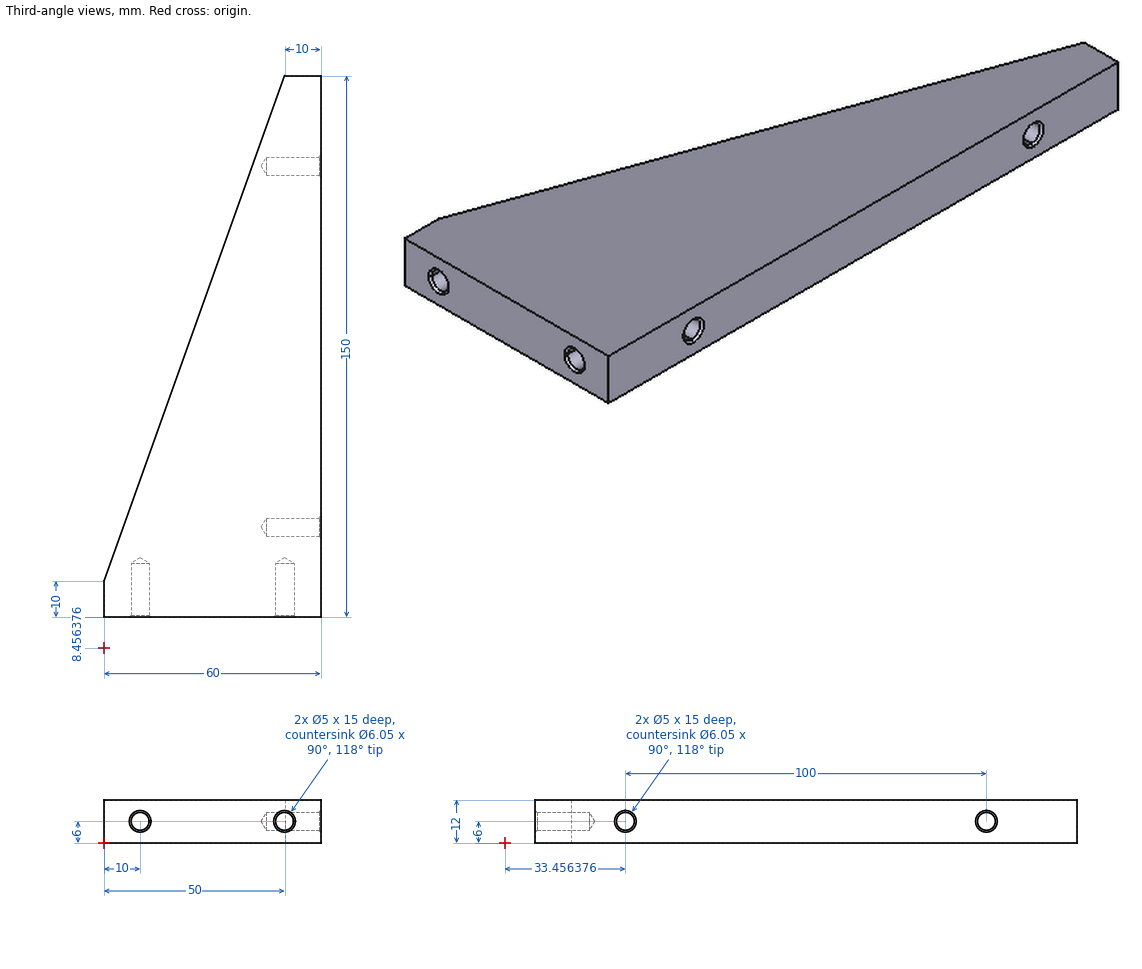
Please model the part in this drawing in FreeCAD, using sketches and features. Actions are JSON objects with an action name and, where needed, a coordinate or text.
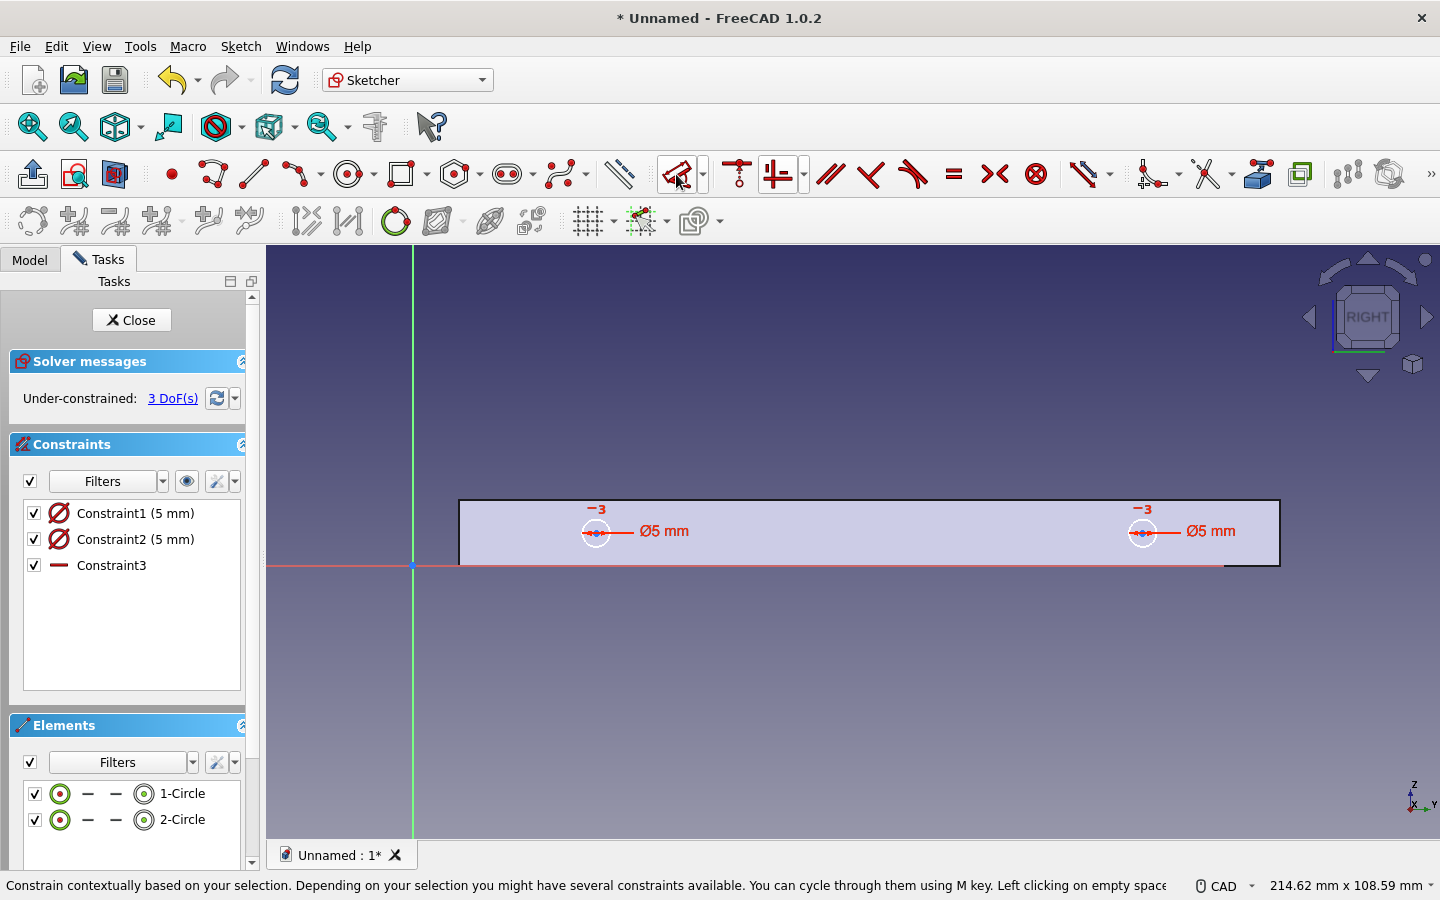
{"action": "left_click", "coordinate": [596, 533]}
{"action": "left_click", "coordinate": [379, 549]}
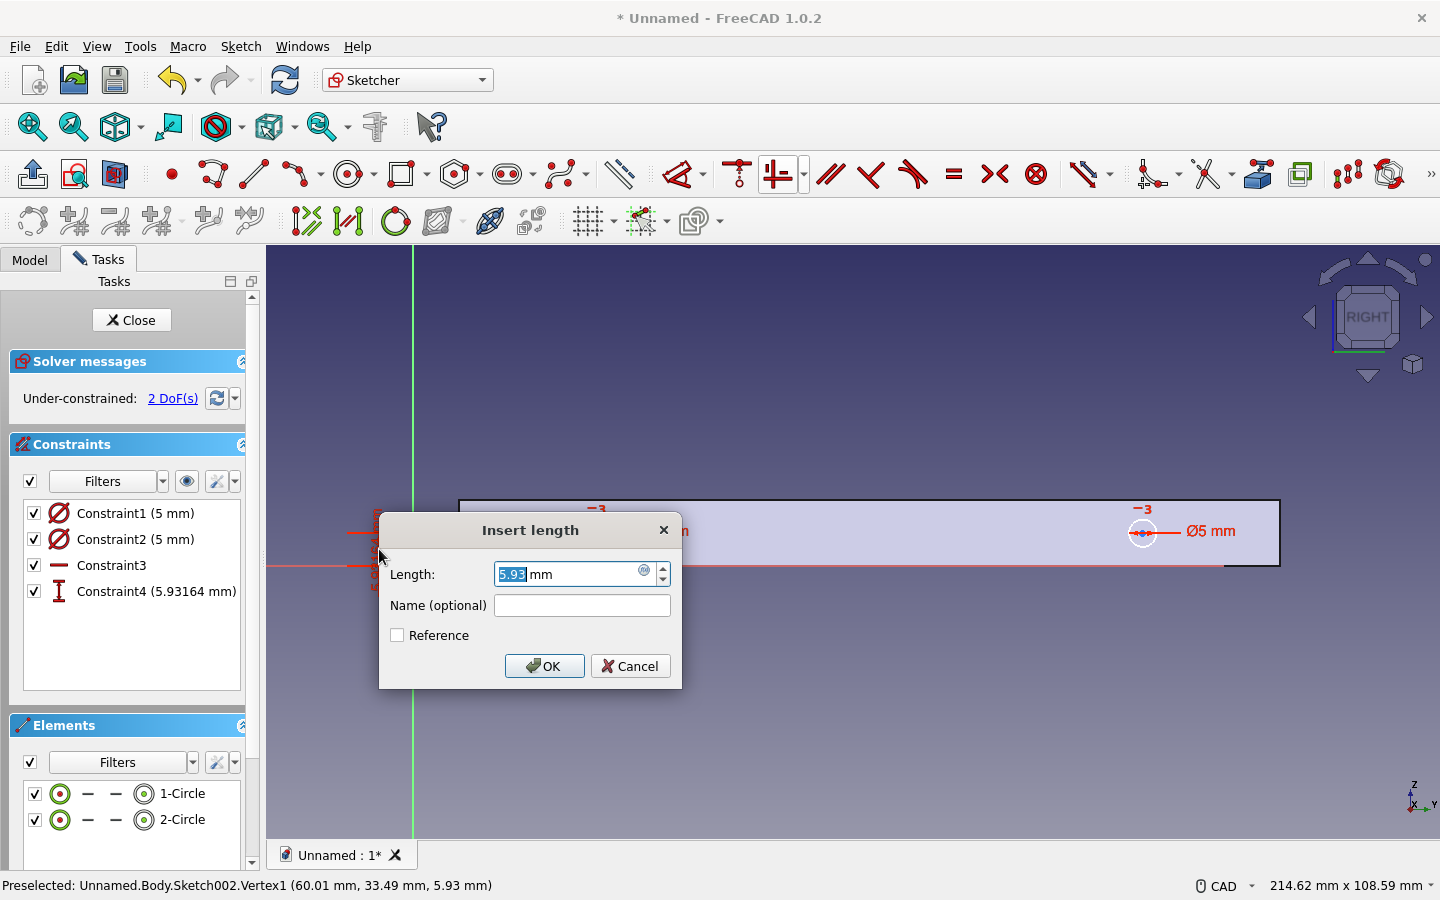
{"action": "type", "text": "6"}
{"action": "key", "text": "Return"}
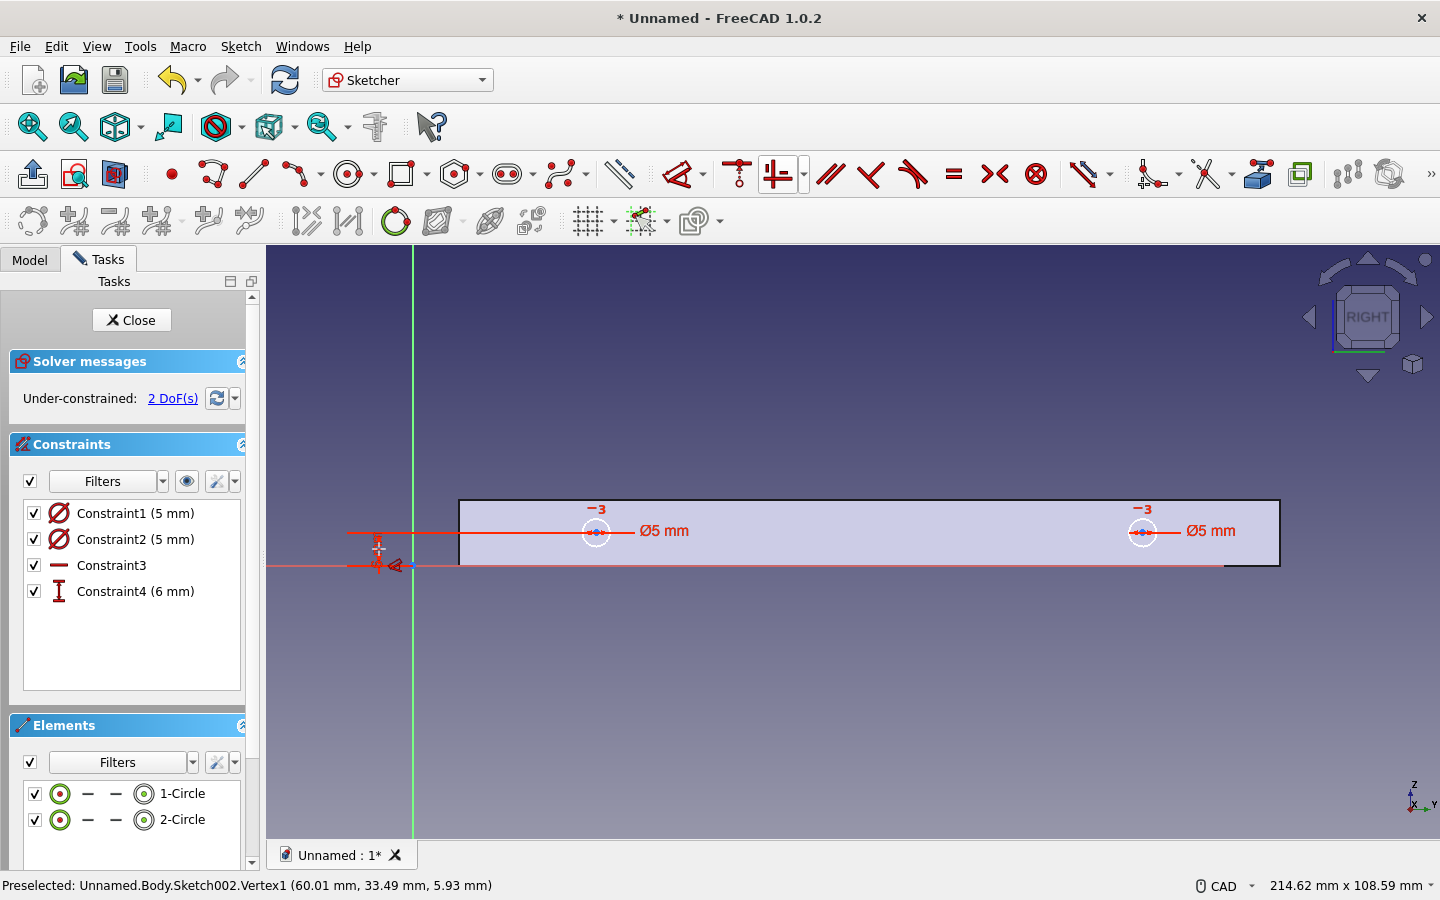
{"action": "left_click", "coordinate": [596, 533]}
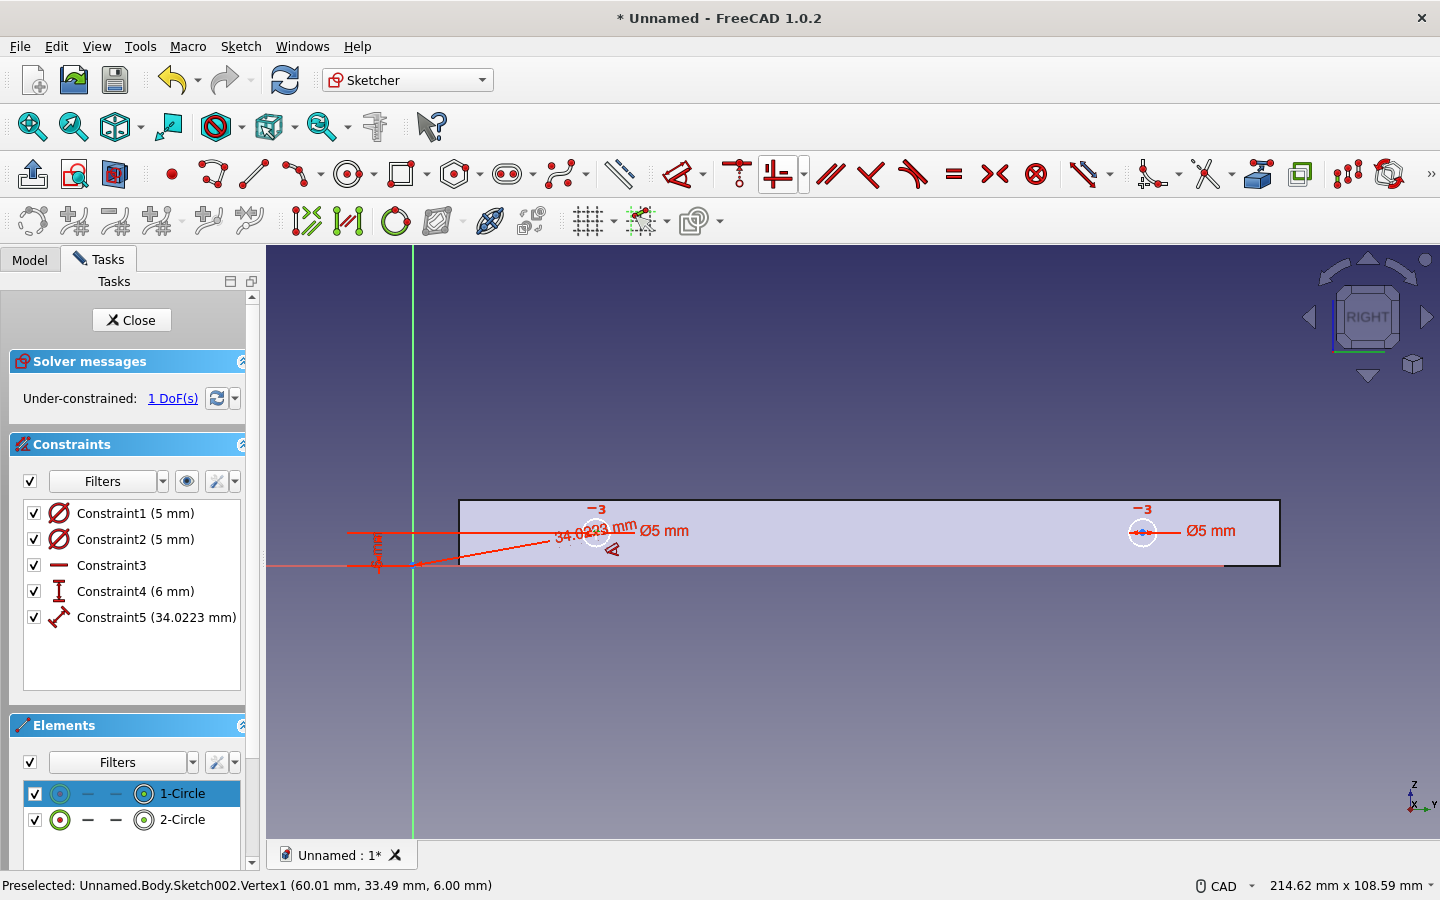
{"action": "left_click", "coordinate": [1143, 533]}
{"action": "left_click", "coordinate": [869, 499]}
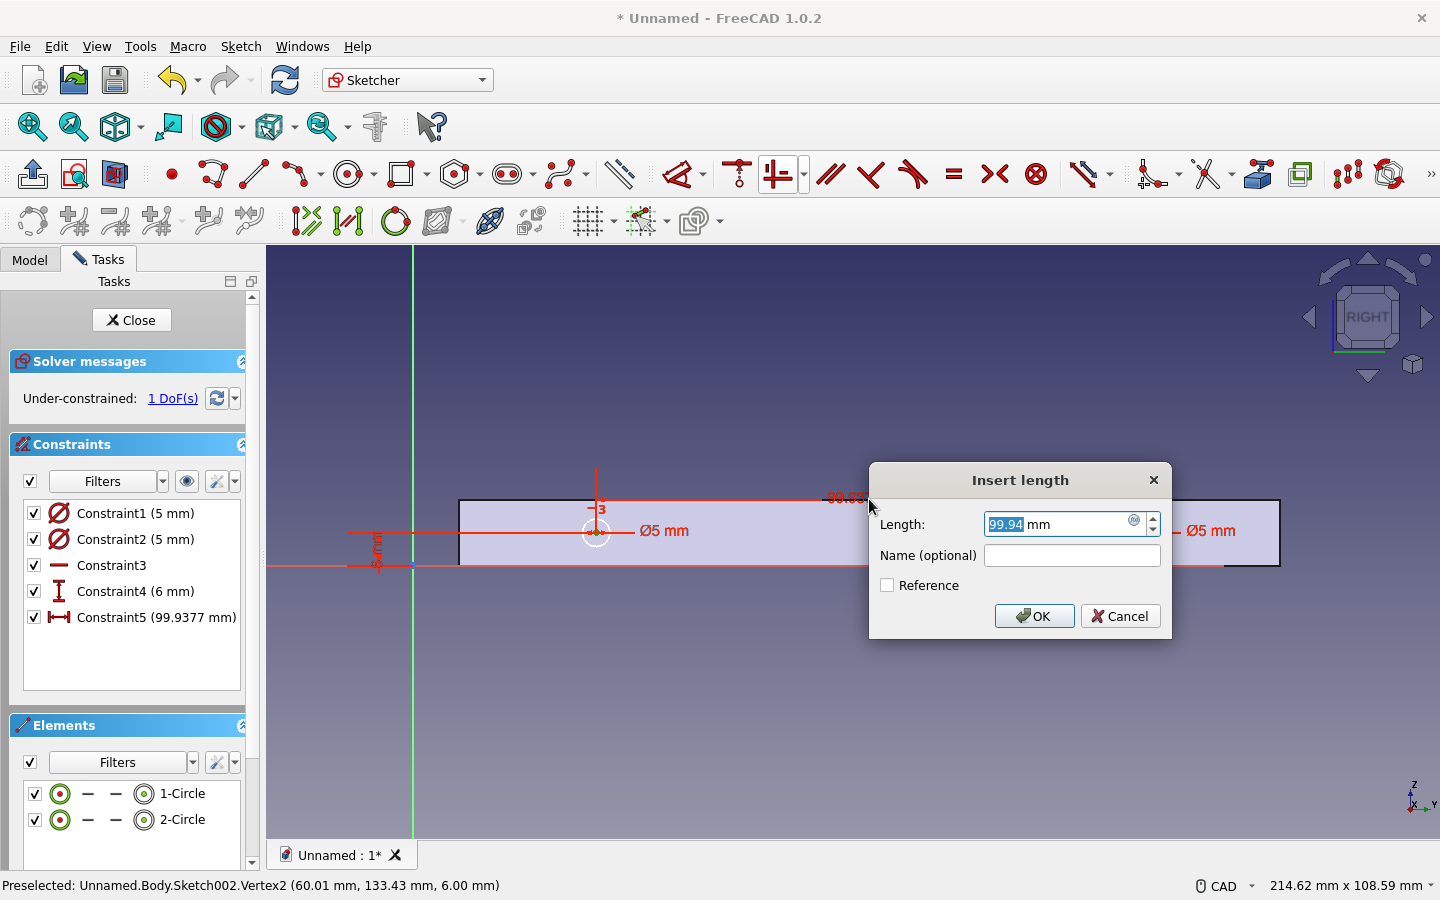
{"action": "type", "text": "100"}
{"action": "key", "text": "Return"}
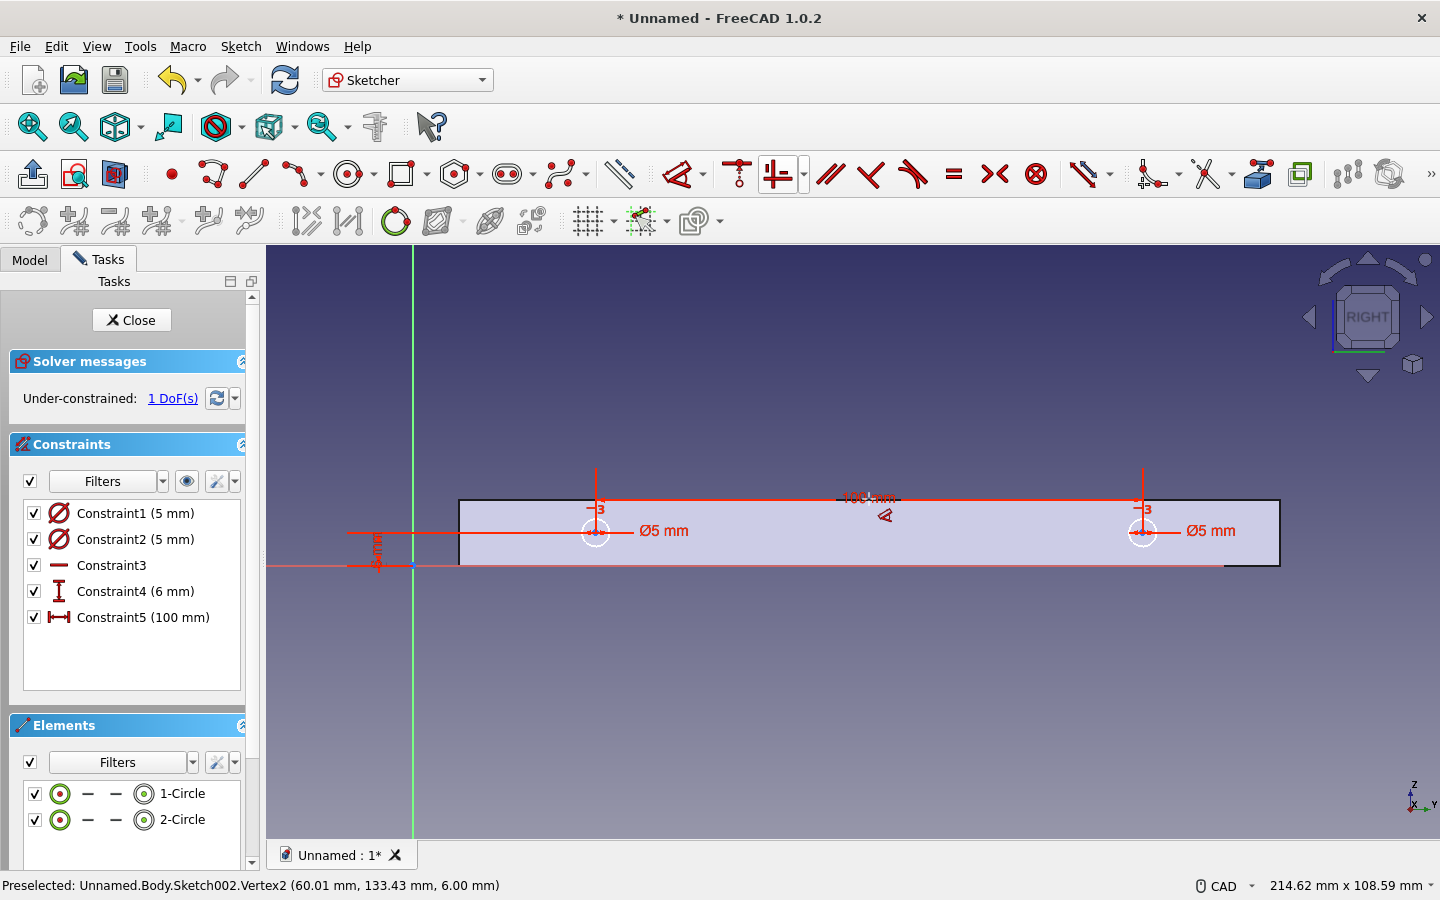
{"action": "left_click", "coordinate": [596, 533]}
{"action": "left_click", "coordinate": [504, 600]}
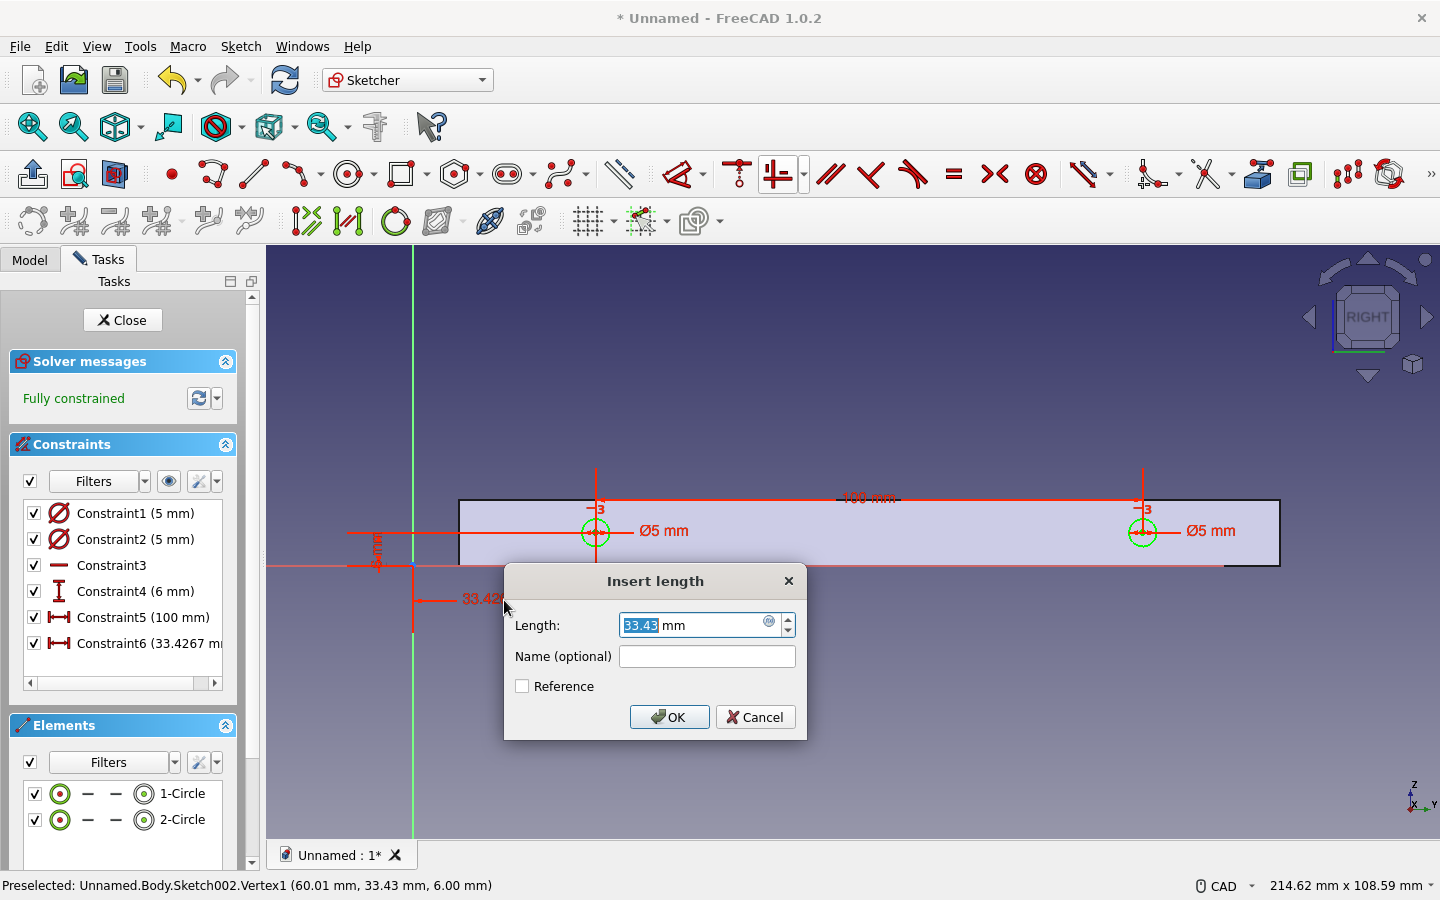
{"action": "type", "text": "33.456376"}
{"action": "key", "text": "Return"}
{"action": "key", "text": "Escape"}